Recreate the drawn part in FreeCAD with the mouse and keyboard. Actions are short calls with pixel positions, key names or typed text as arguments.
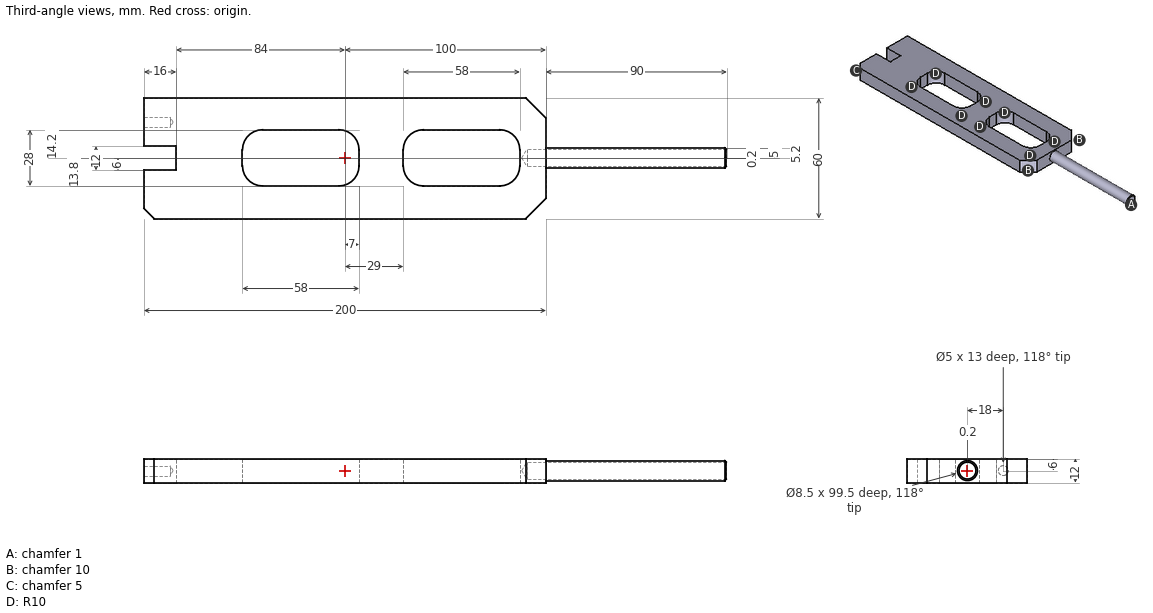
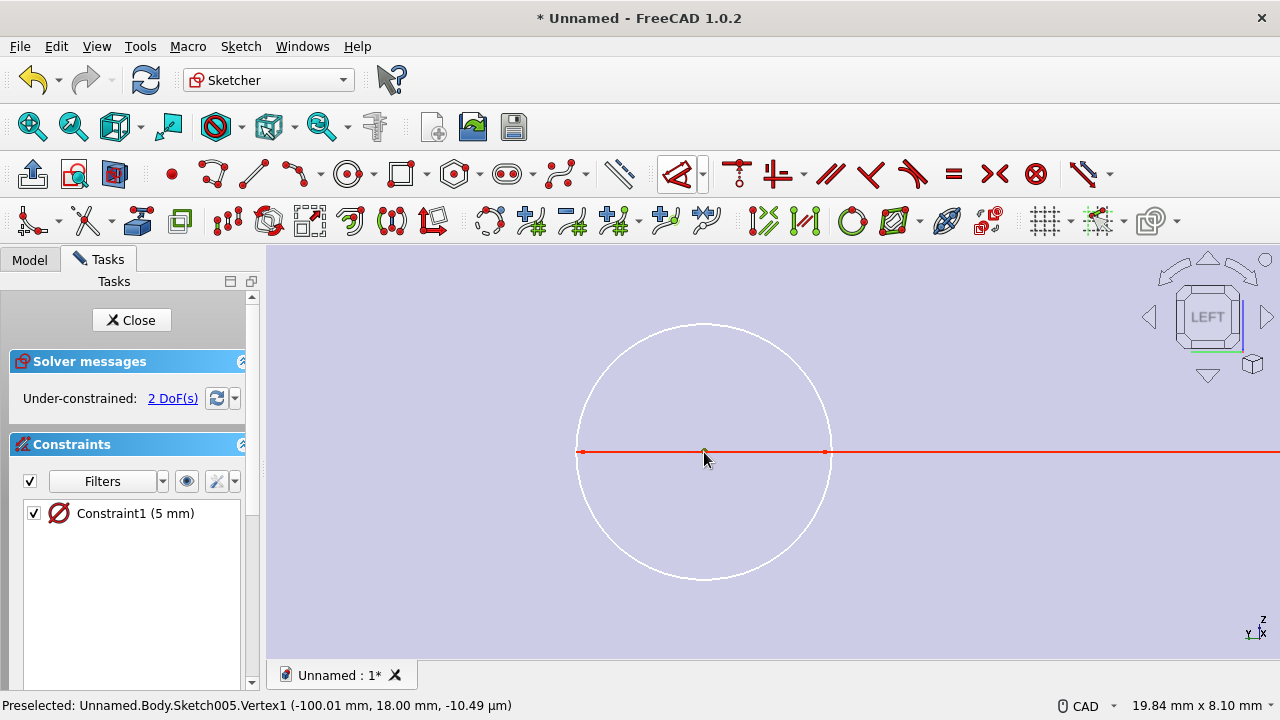
key(i)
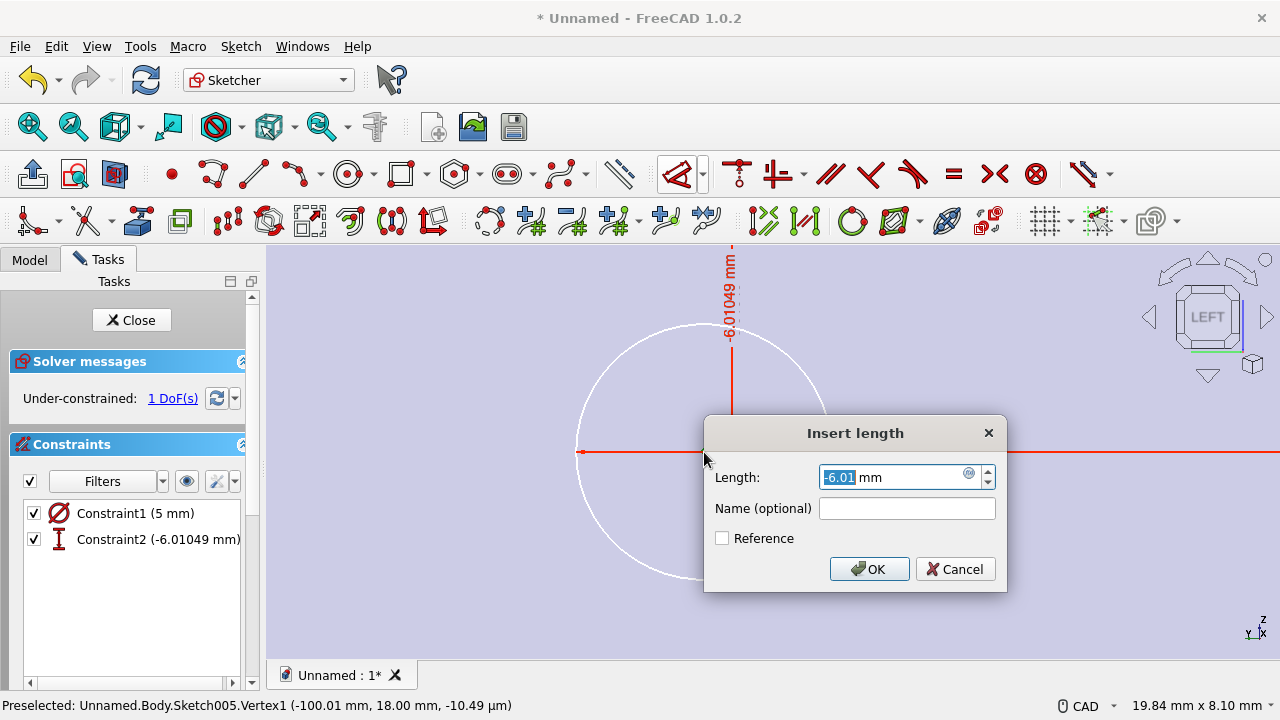
text(-6)
key(Return)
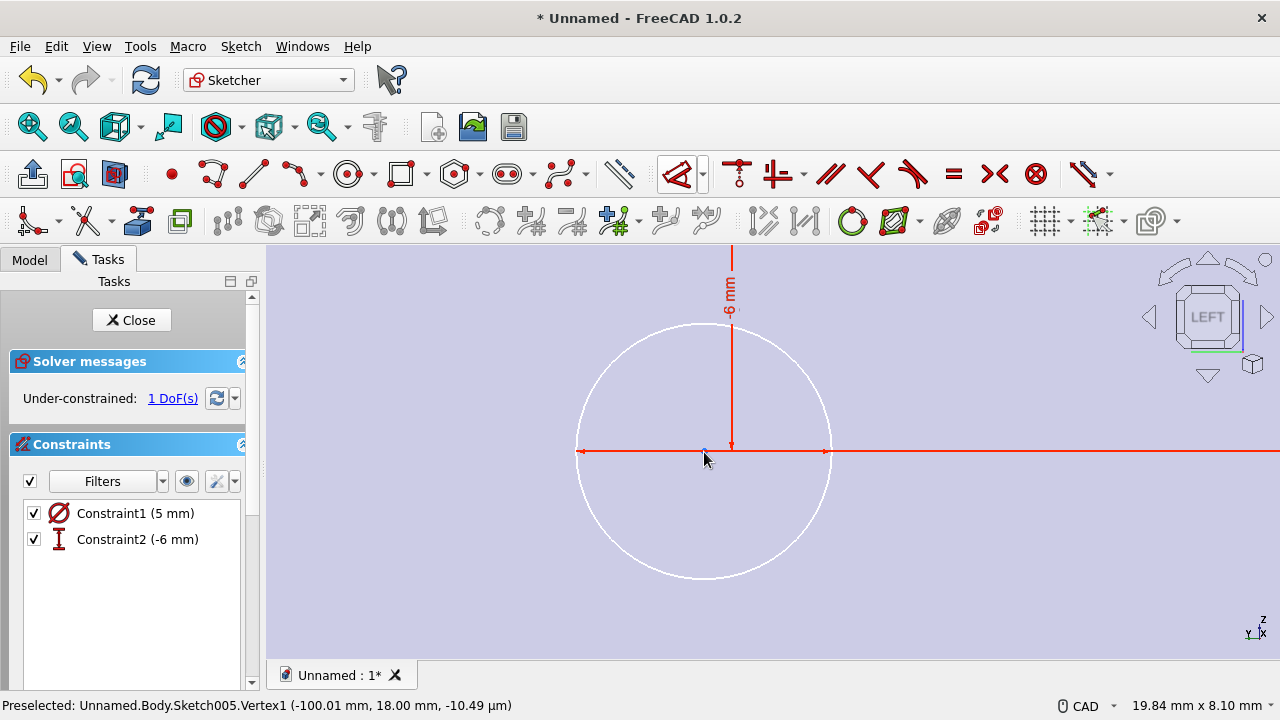
click(704, 451)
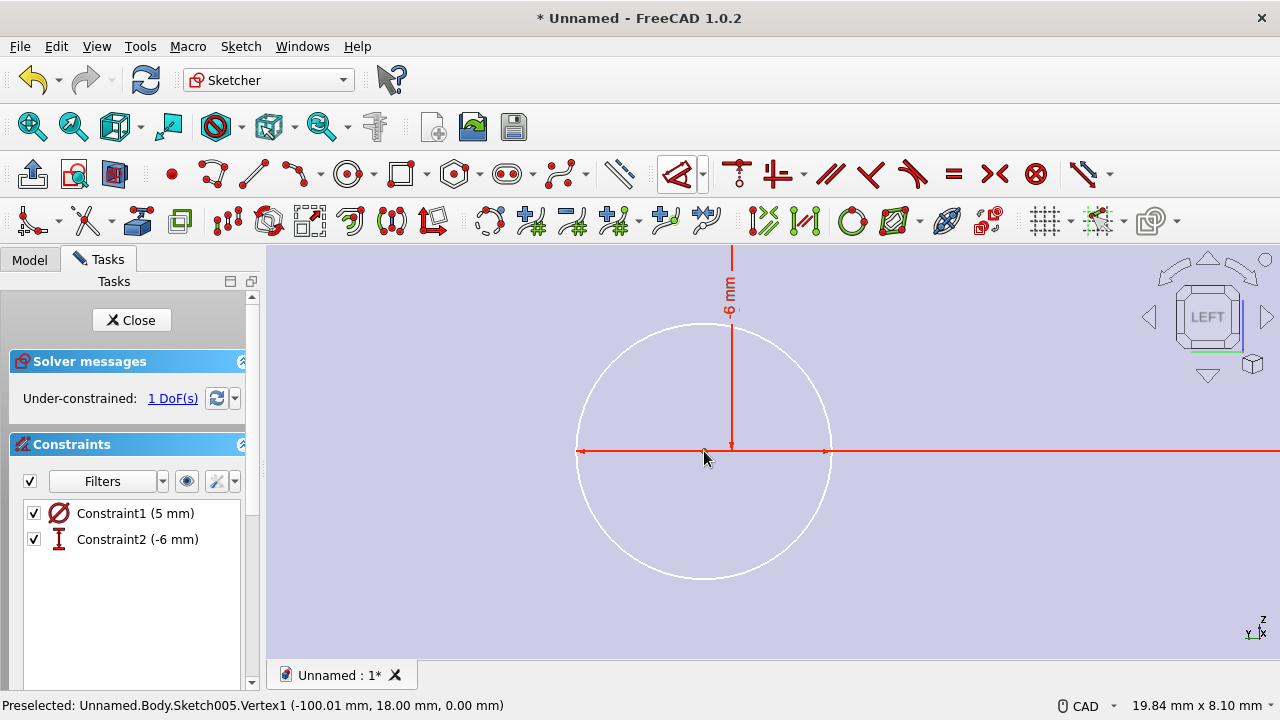
key(l)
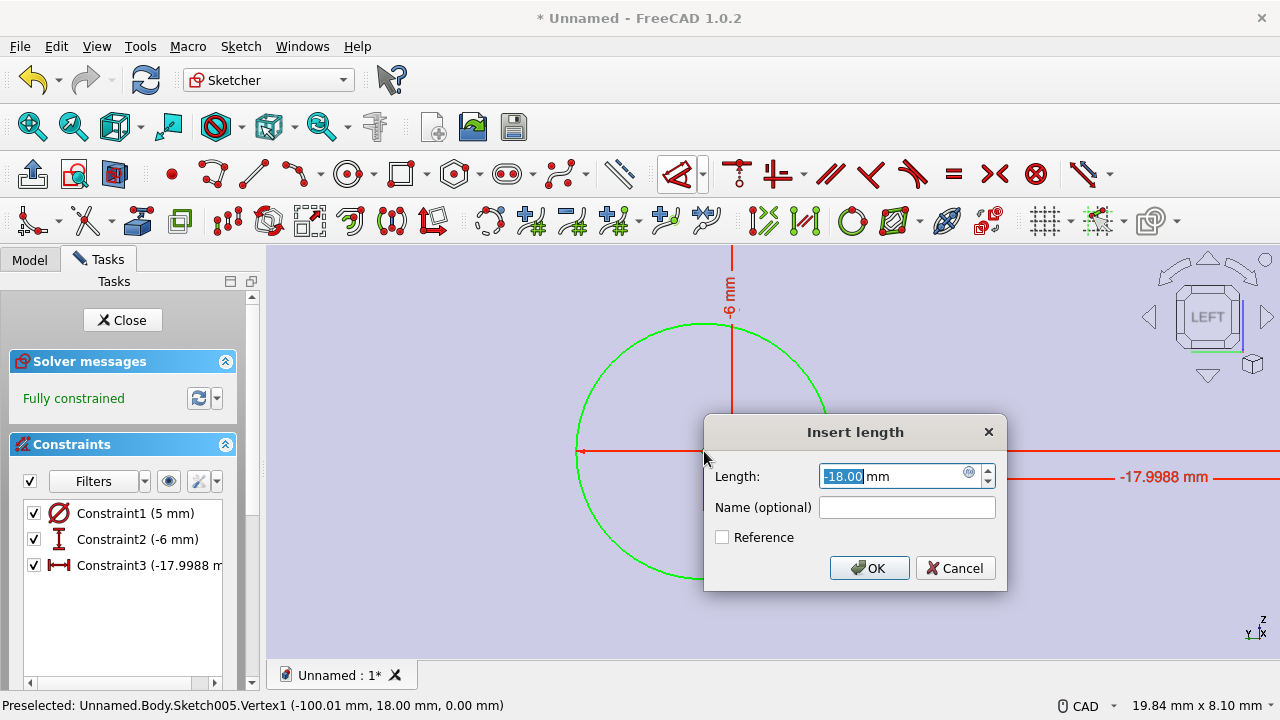
text(-18)
key(Return)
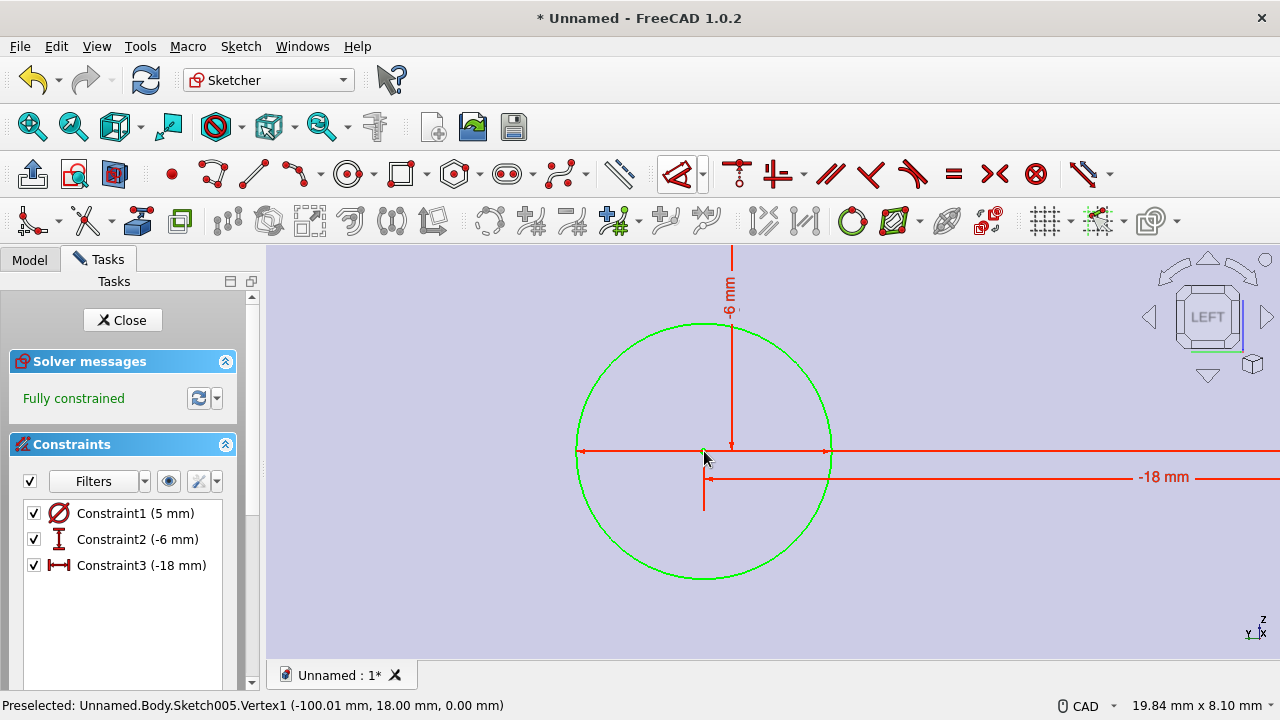
click(123, 320)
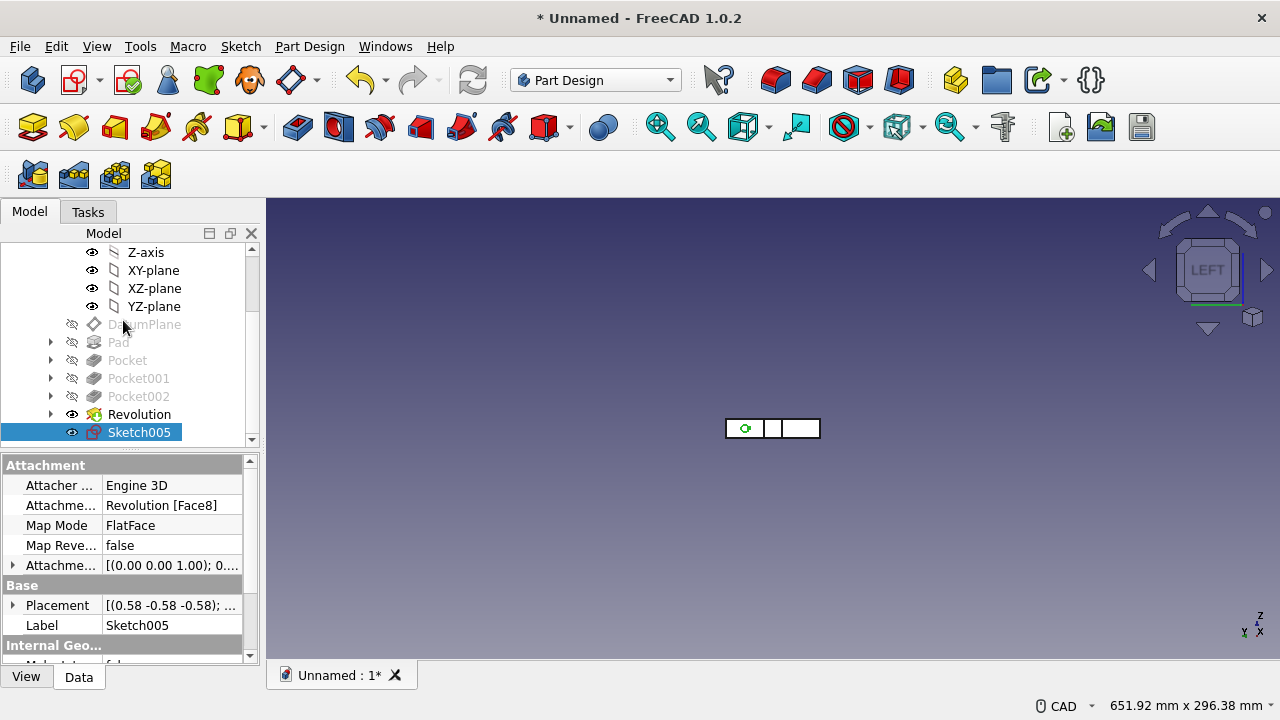
click(339, 128)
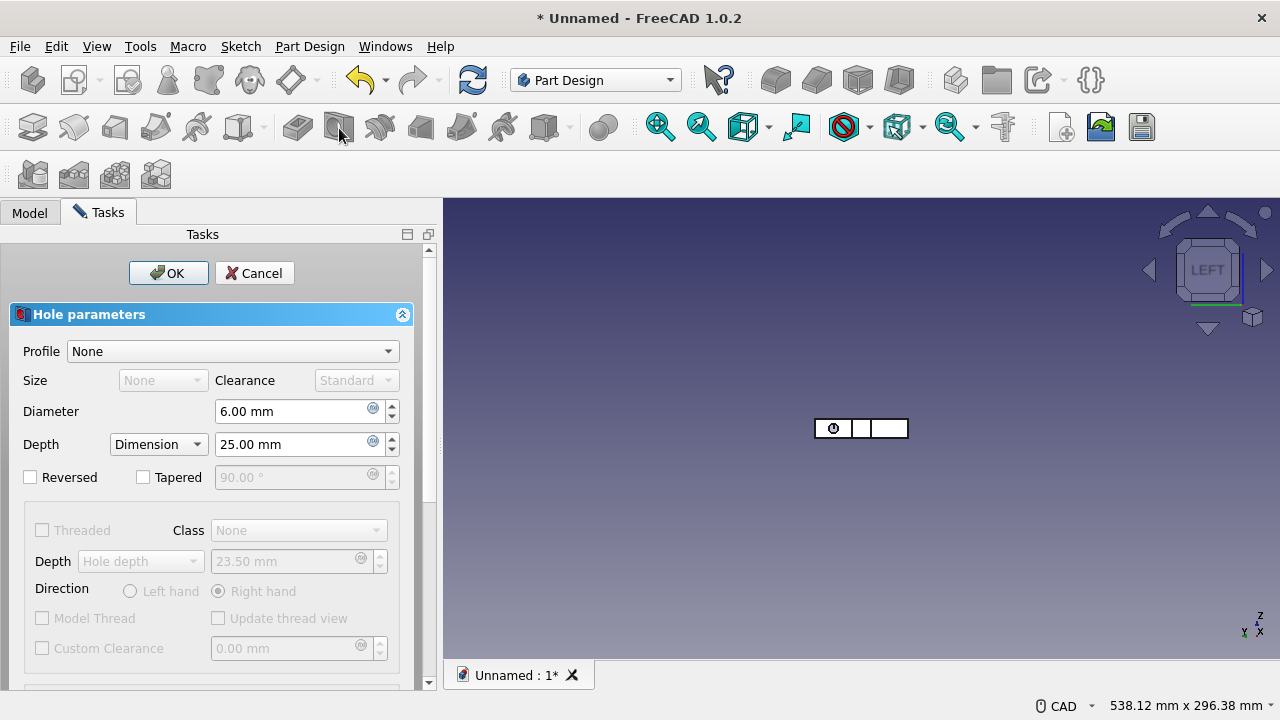
triple_click(300, 412)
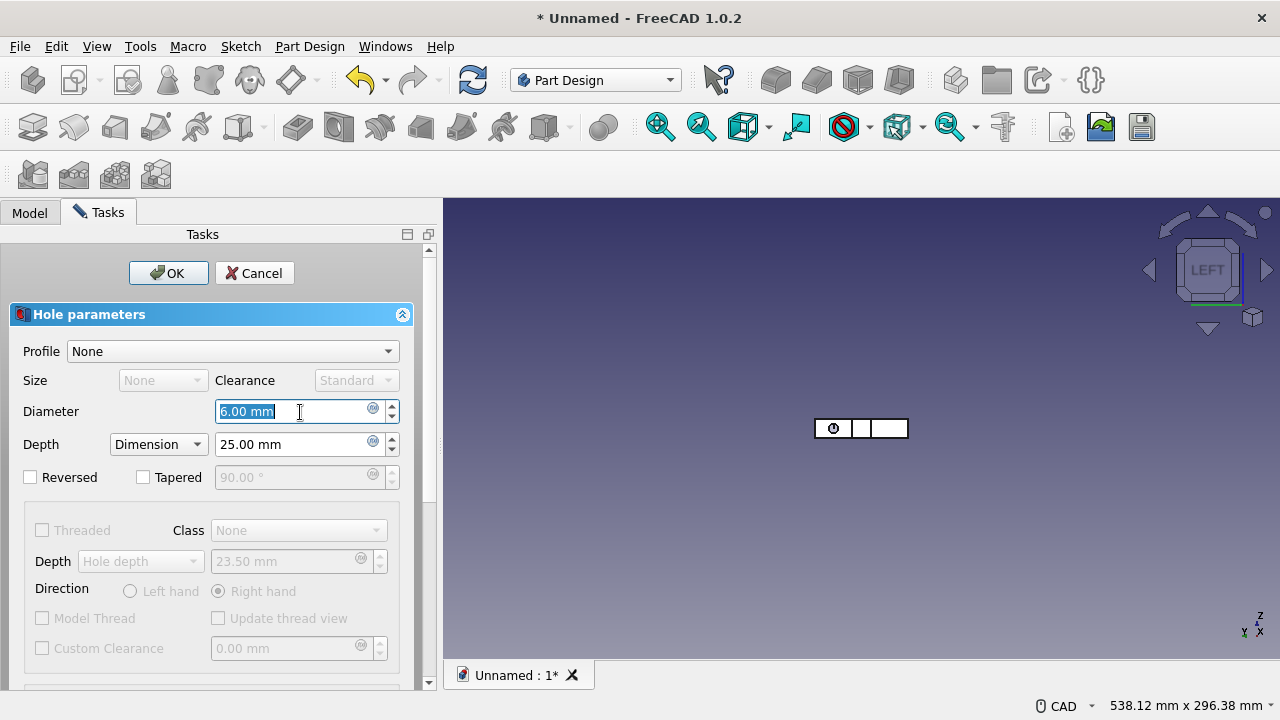
text(5)
key(Tab)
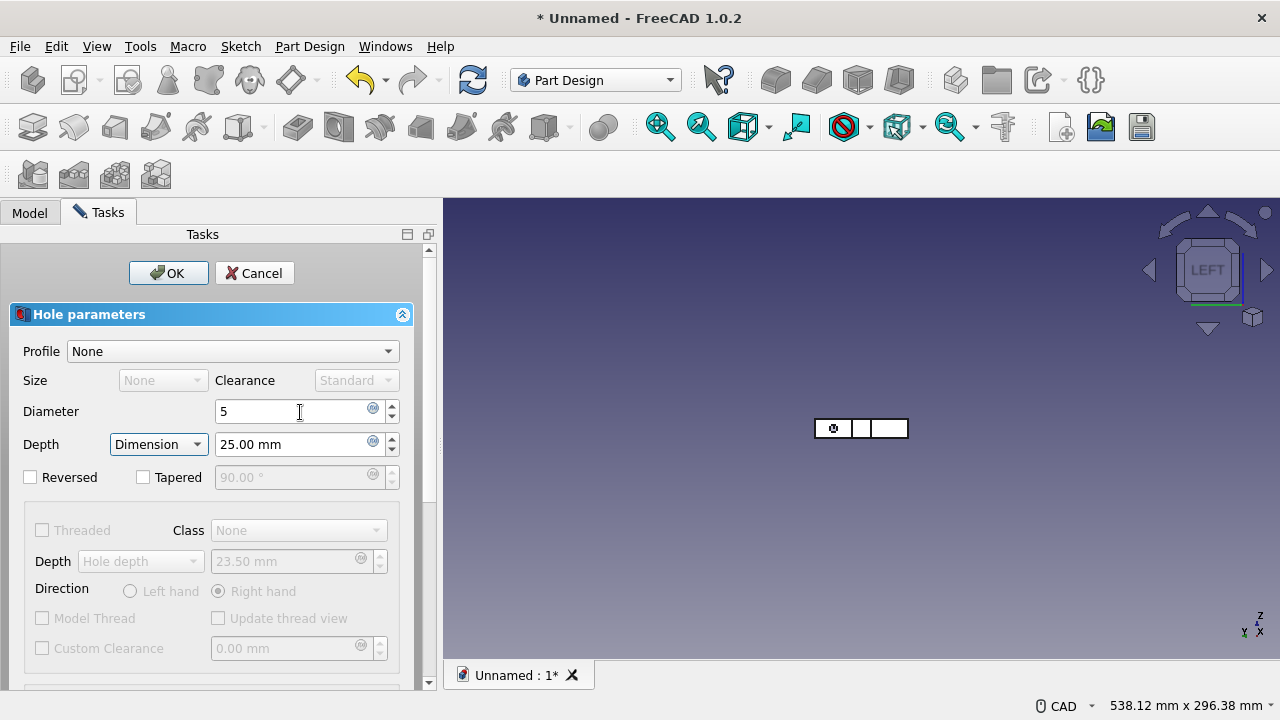
triple_click(300, 444)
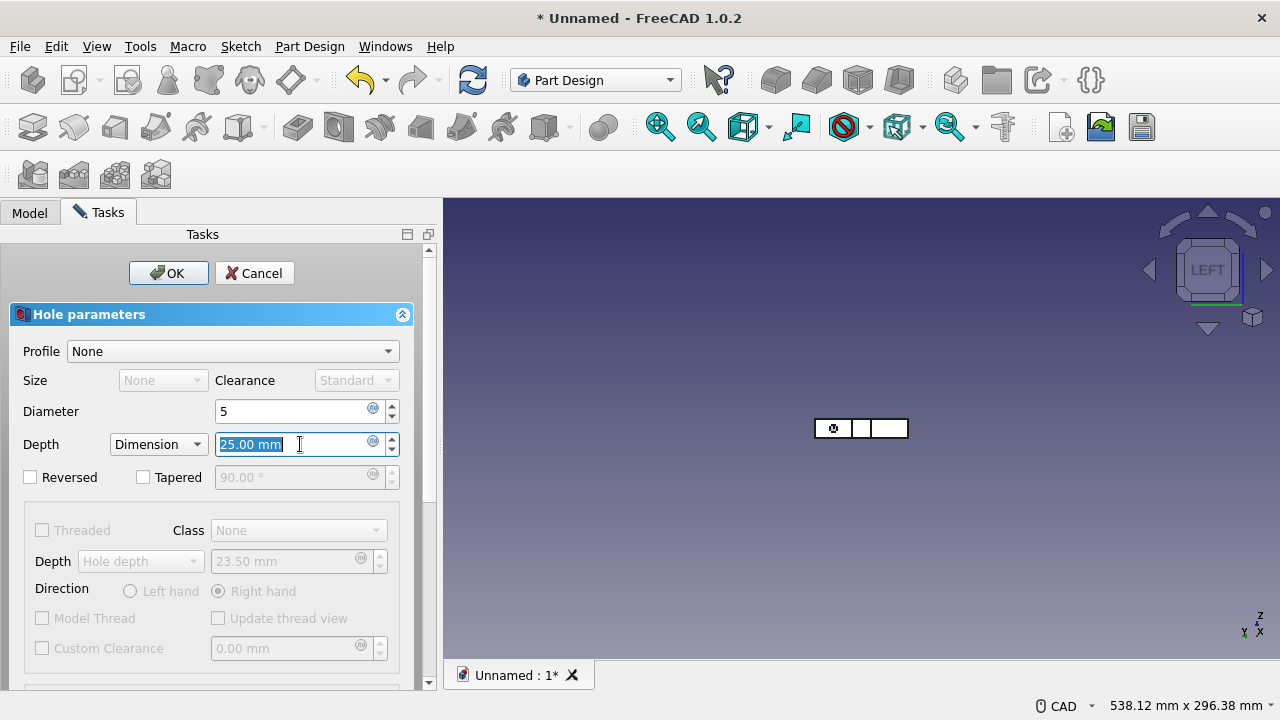
text(13)
key(Tab)